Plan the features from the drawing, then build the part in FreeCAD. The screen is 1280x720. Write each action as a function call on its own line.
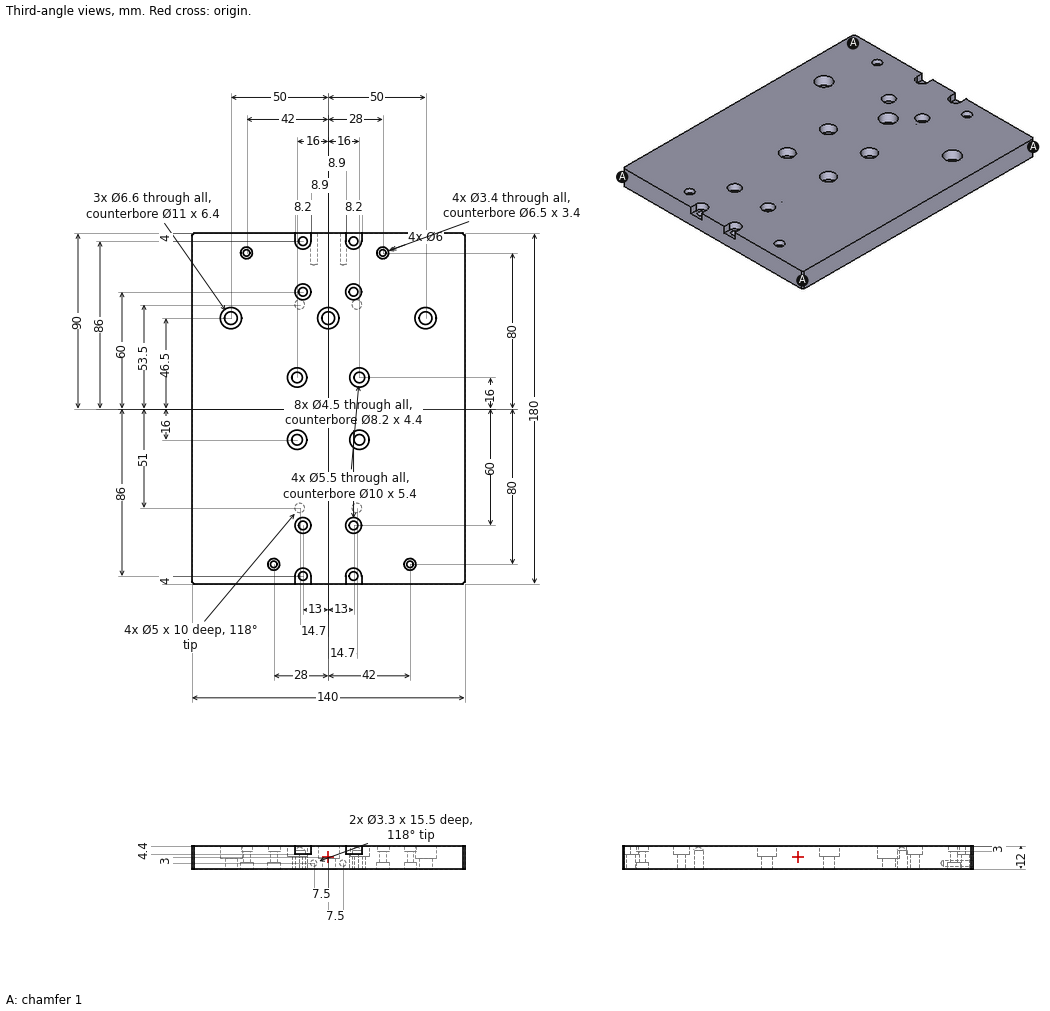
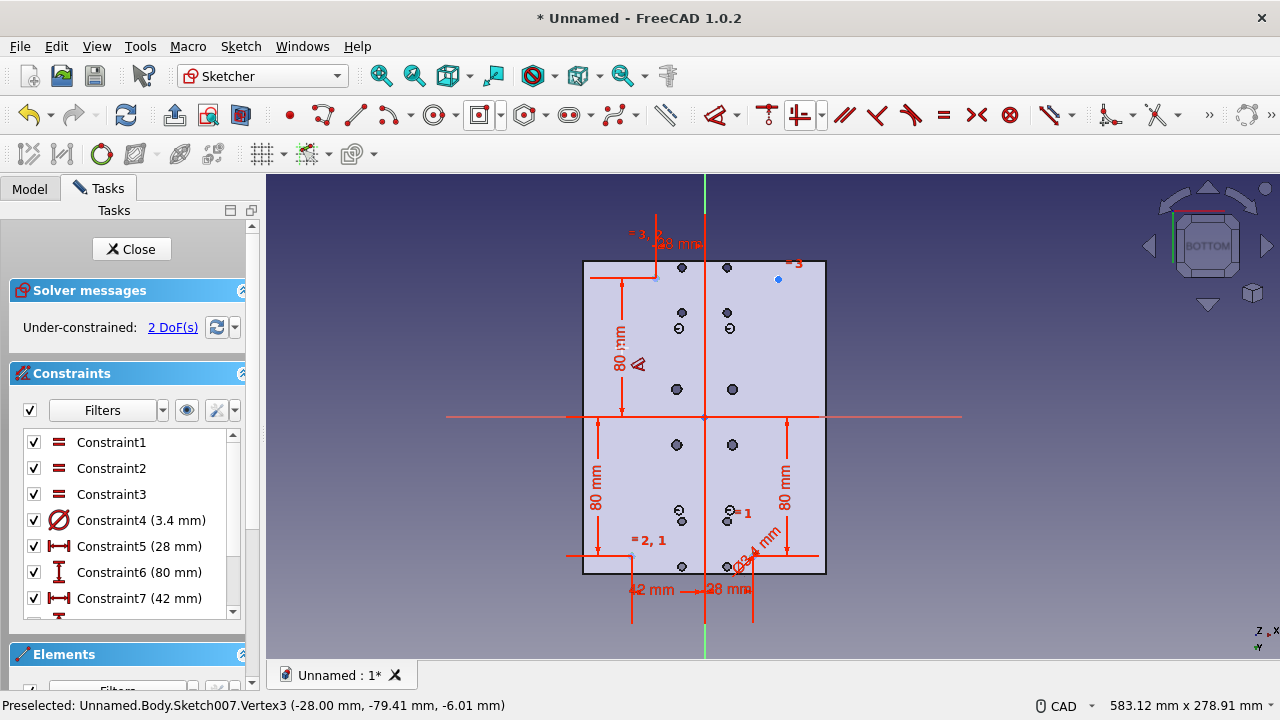
click(778, 279)
click(758, 245)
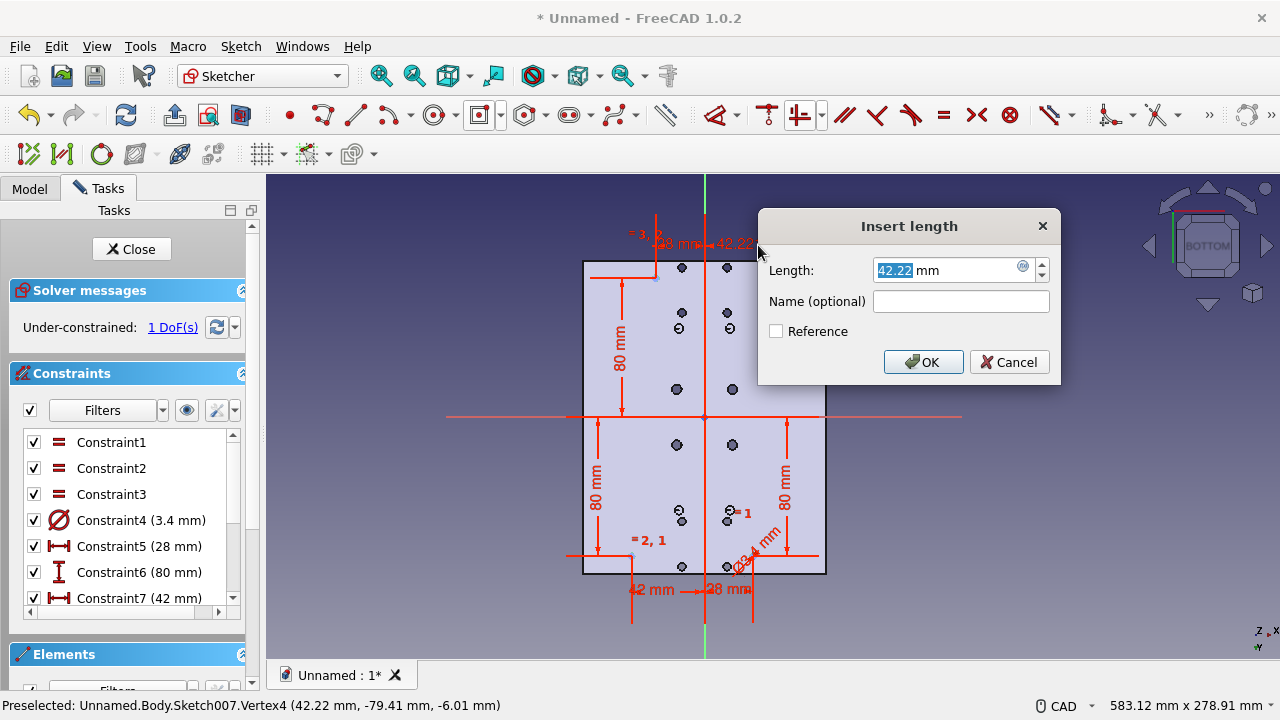
text(42)
key(Return)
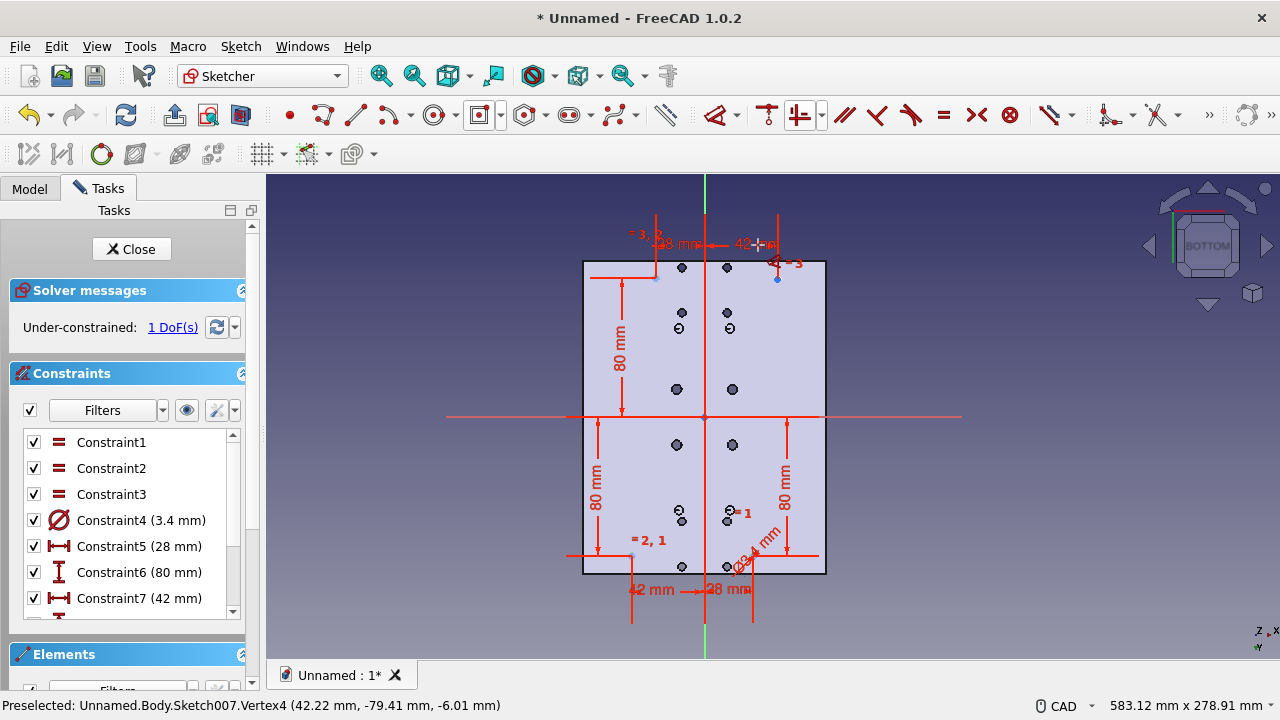
click(778, 279)
click(812, 348)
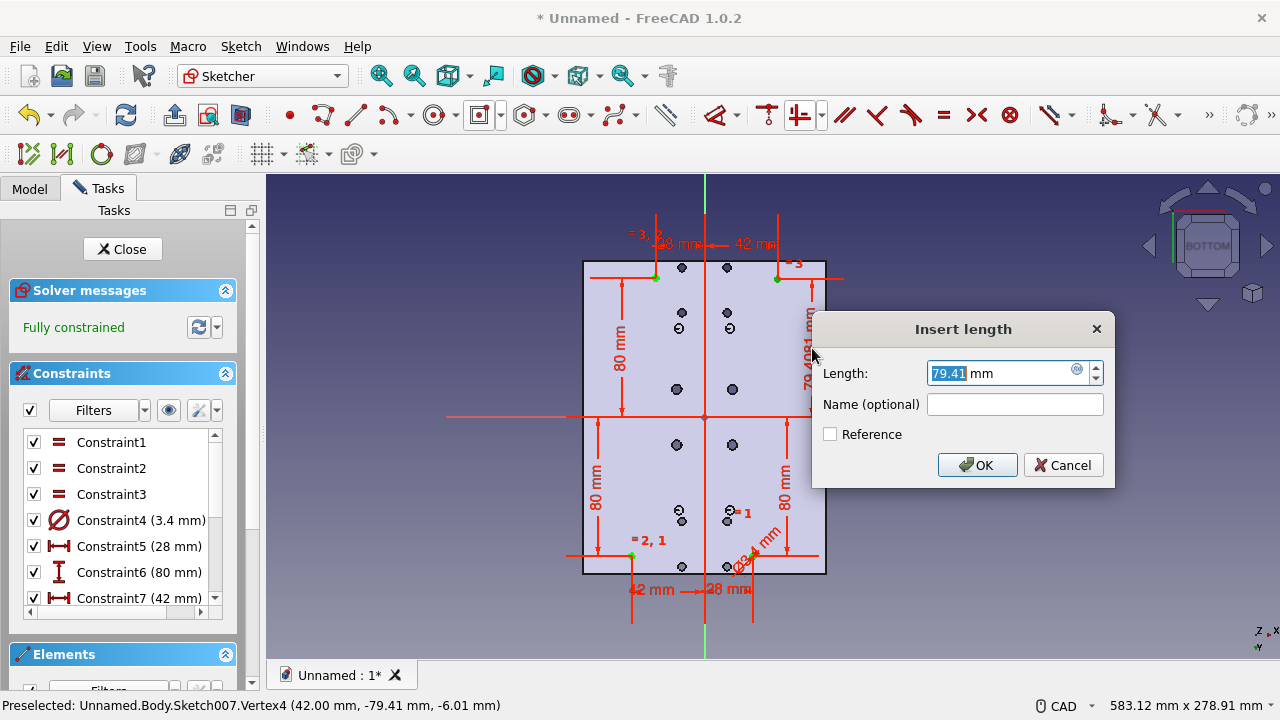
text(80)
key(Return)
key(Escape)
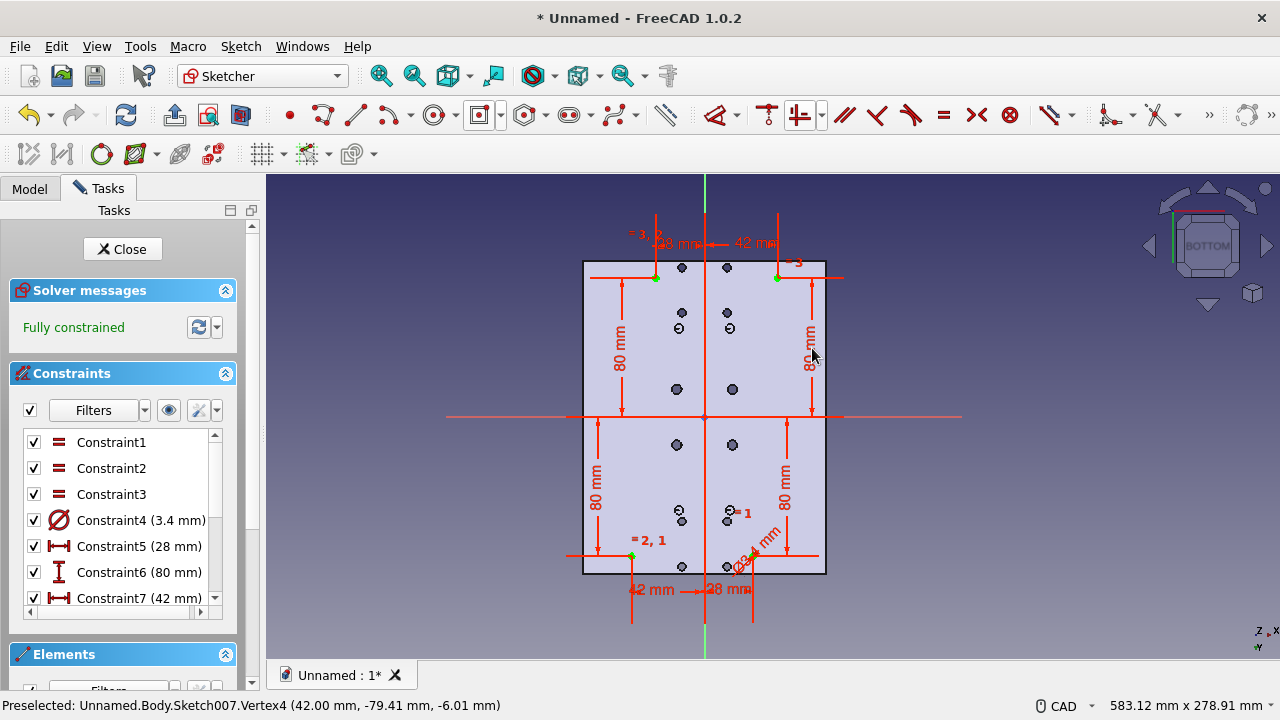
click(123, 249)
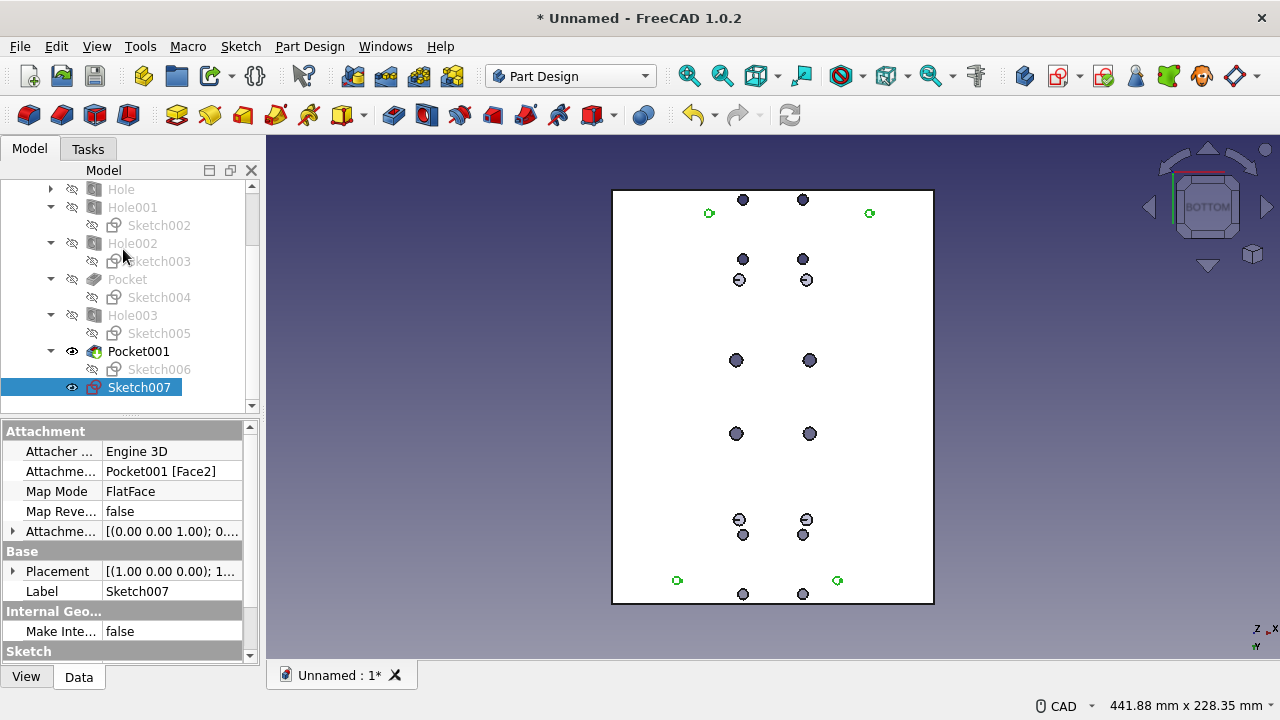
click(427, 116)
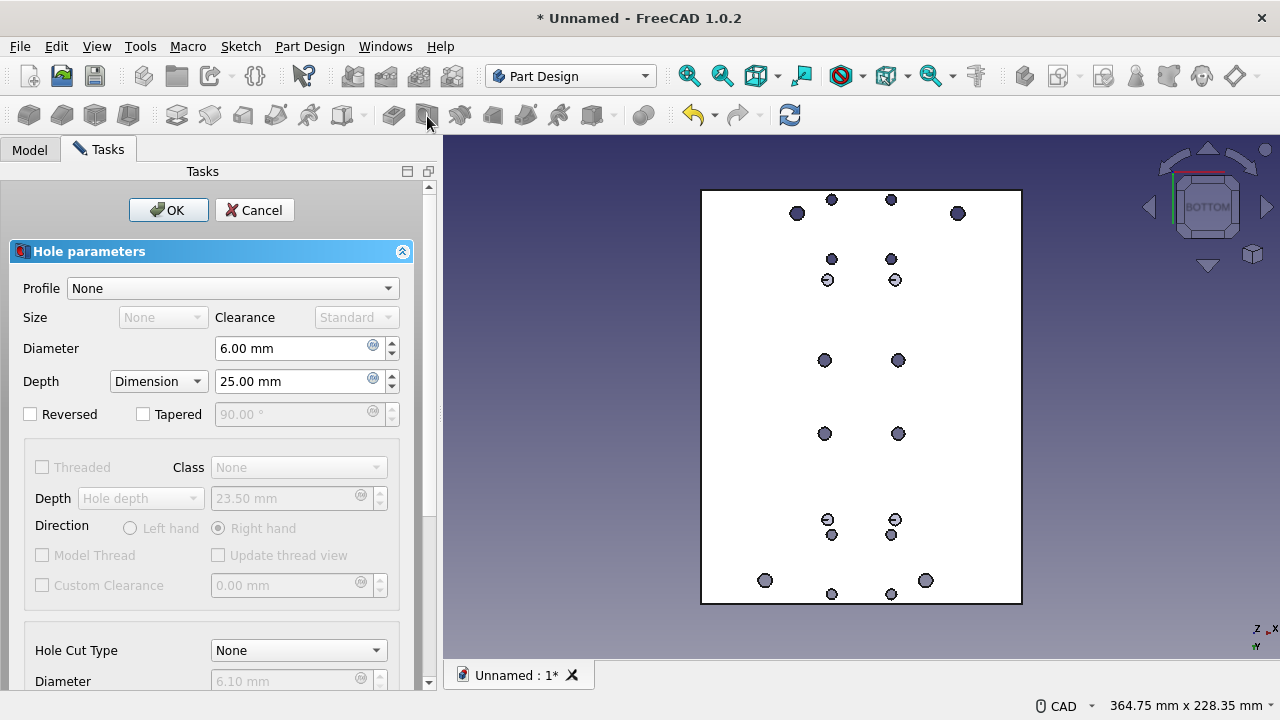
triple_click(300, 348)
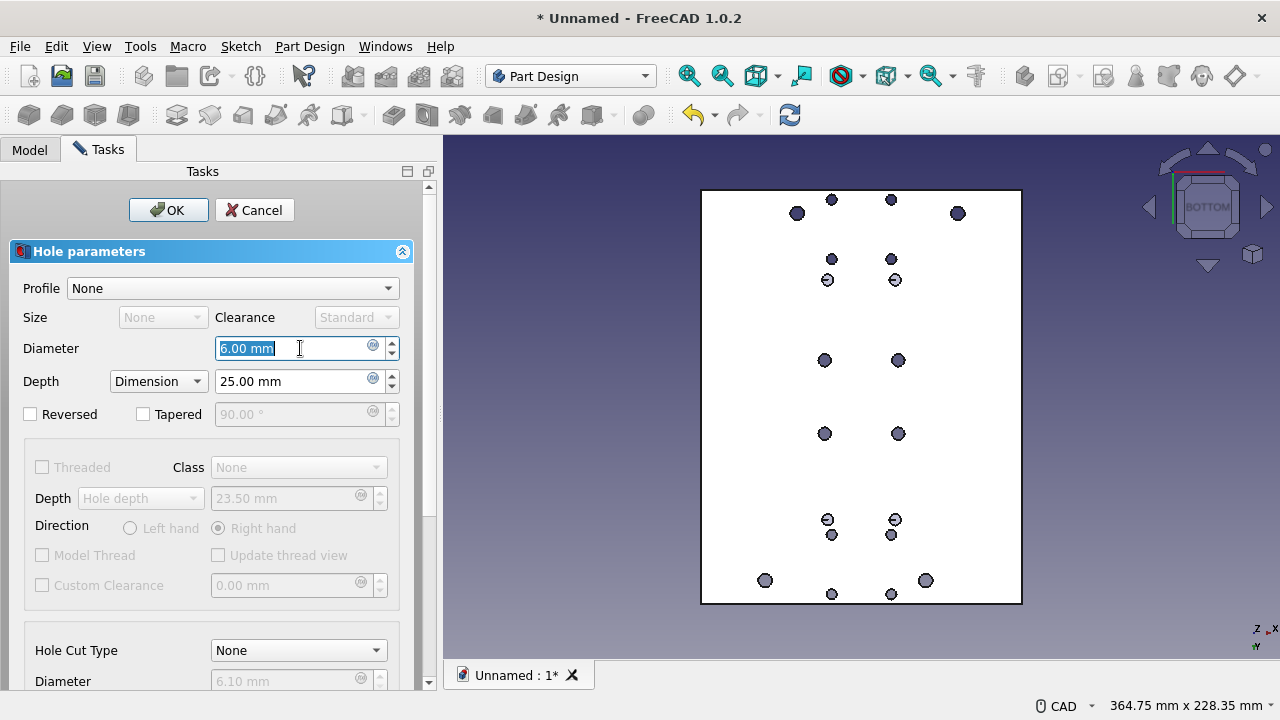
text(3.4)
key(Tab)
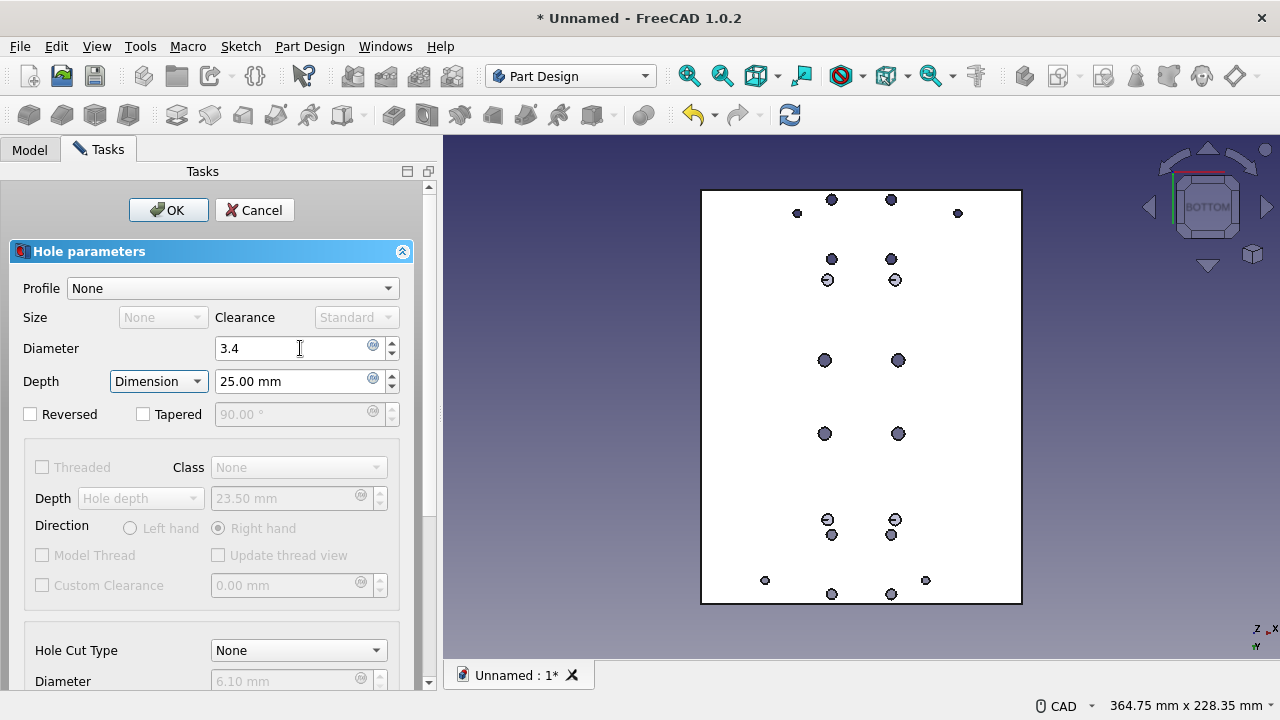
click(160, 382)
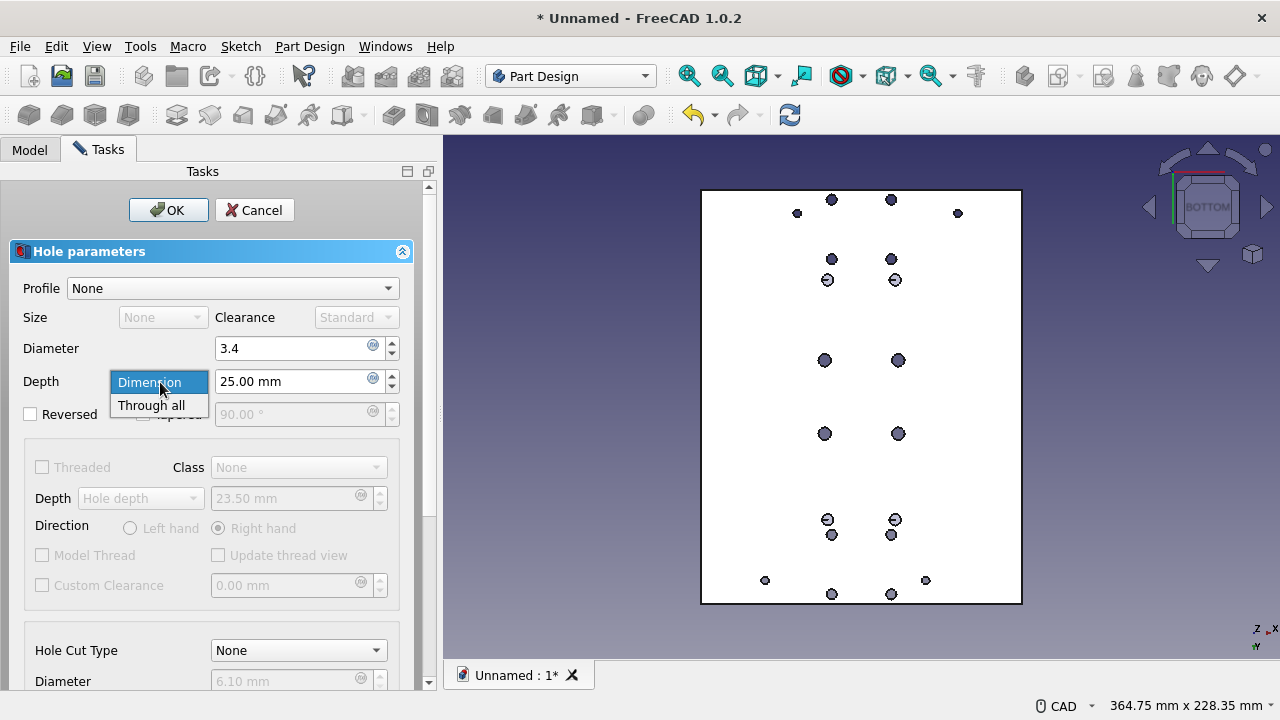
click(158, 406)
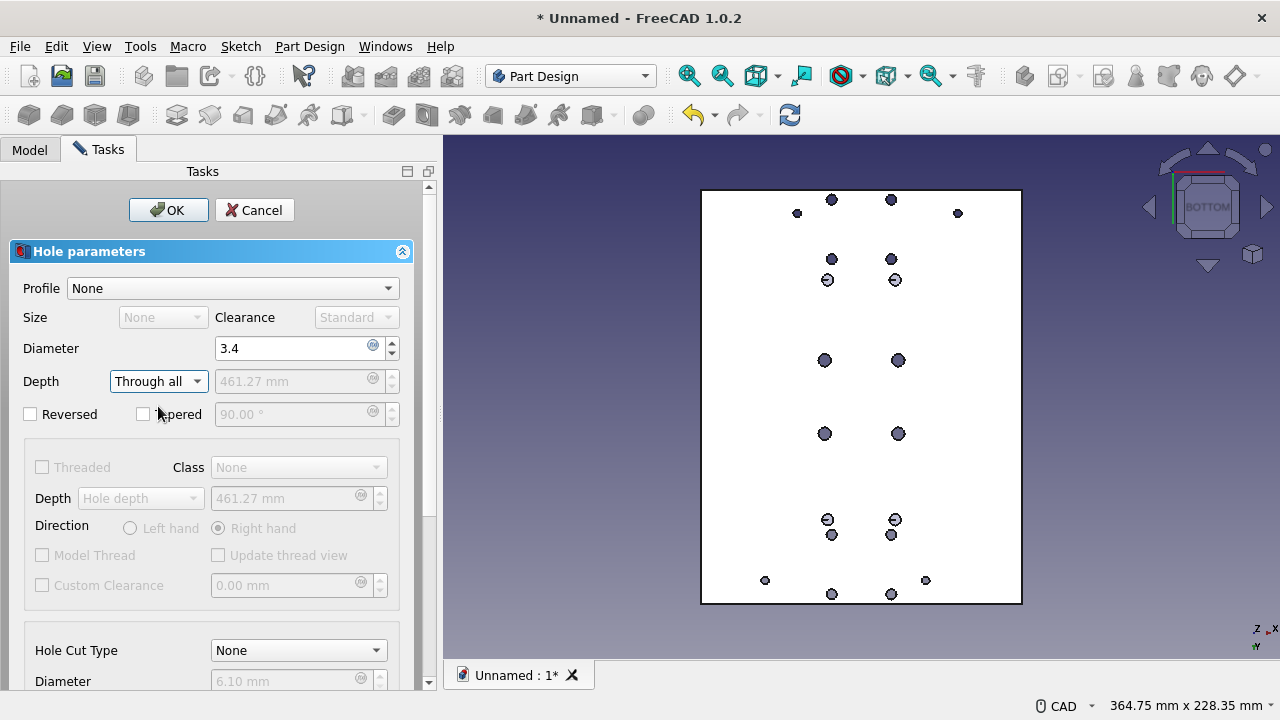
click(300, 650)